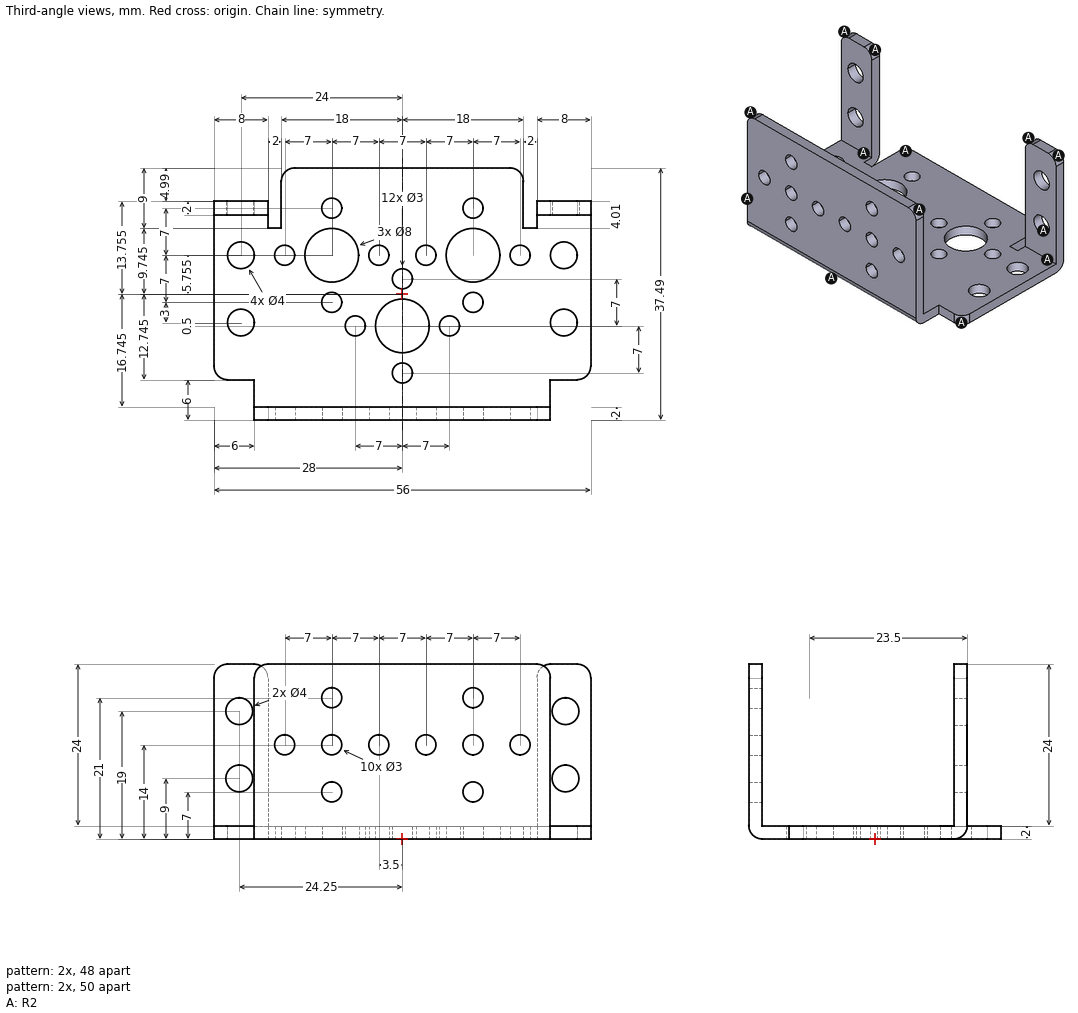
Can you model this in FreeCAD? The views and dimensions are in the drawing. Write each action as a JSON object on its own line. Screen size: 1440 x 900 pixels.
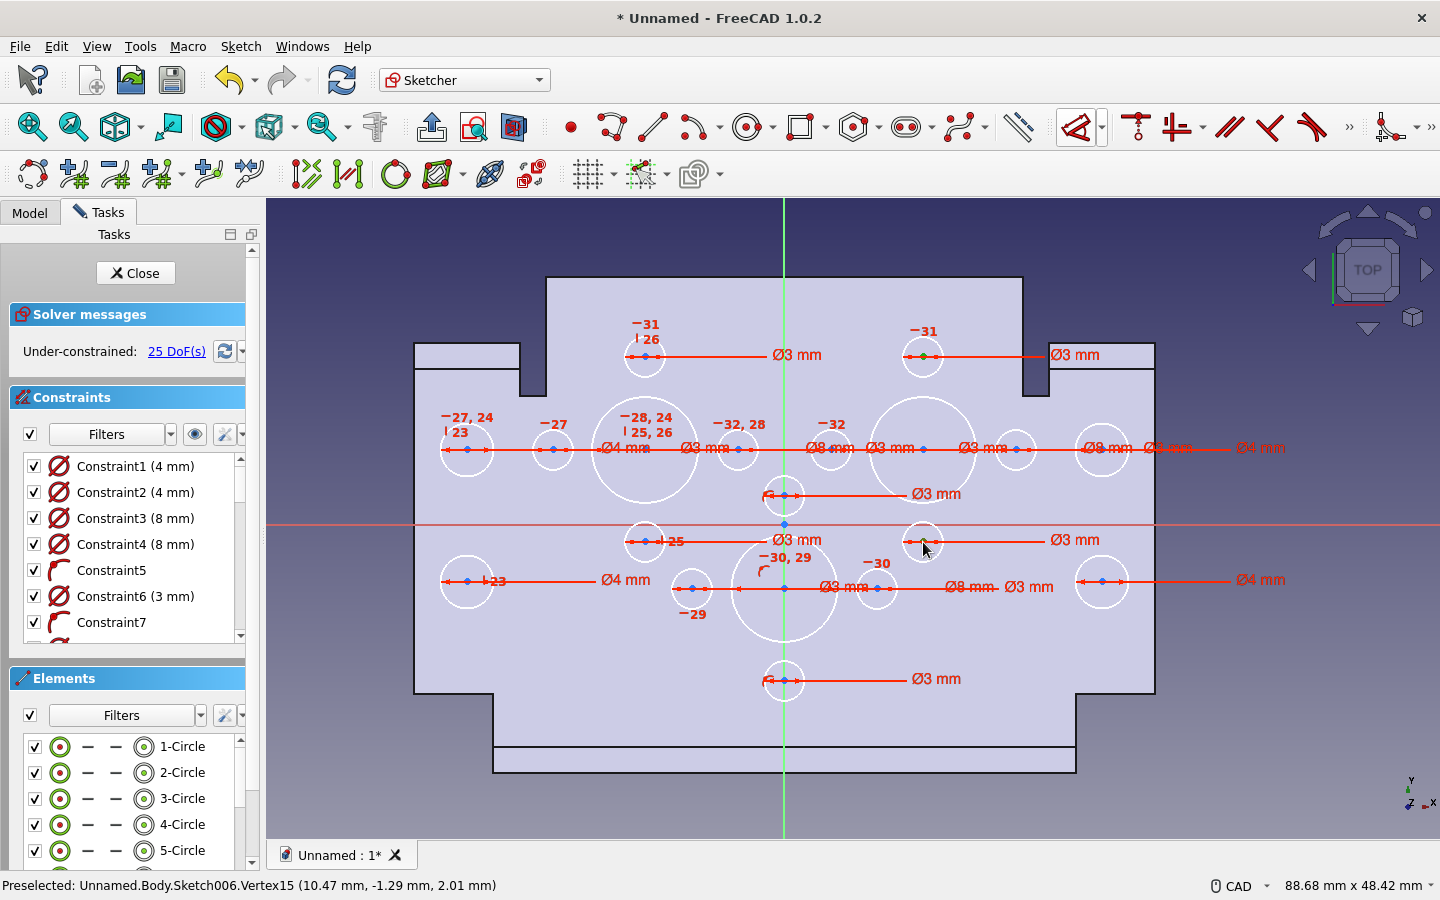
{"action": "key", "text": "v"}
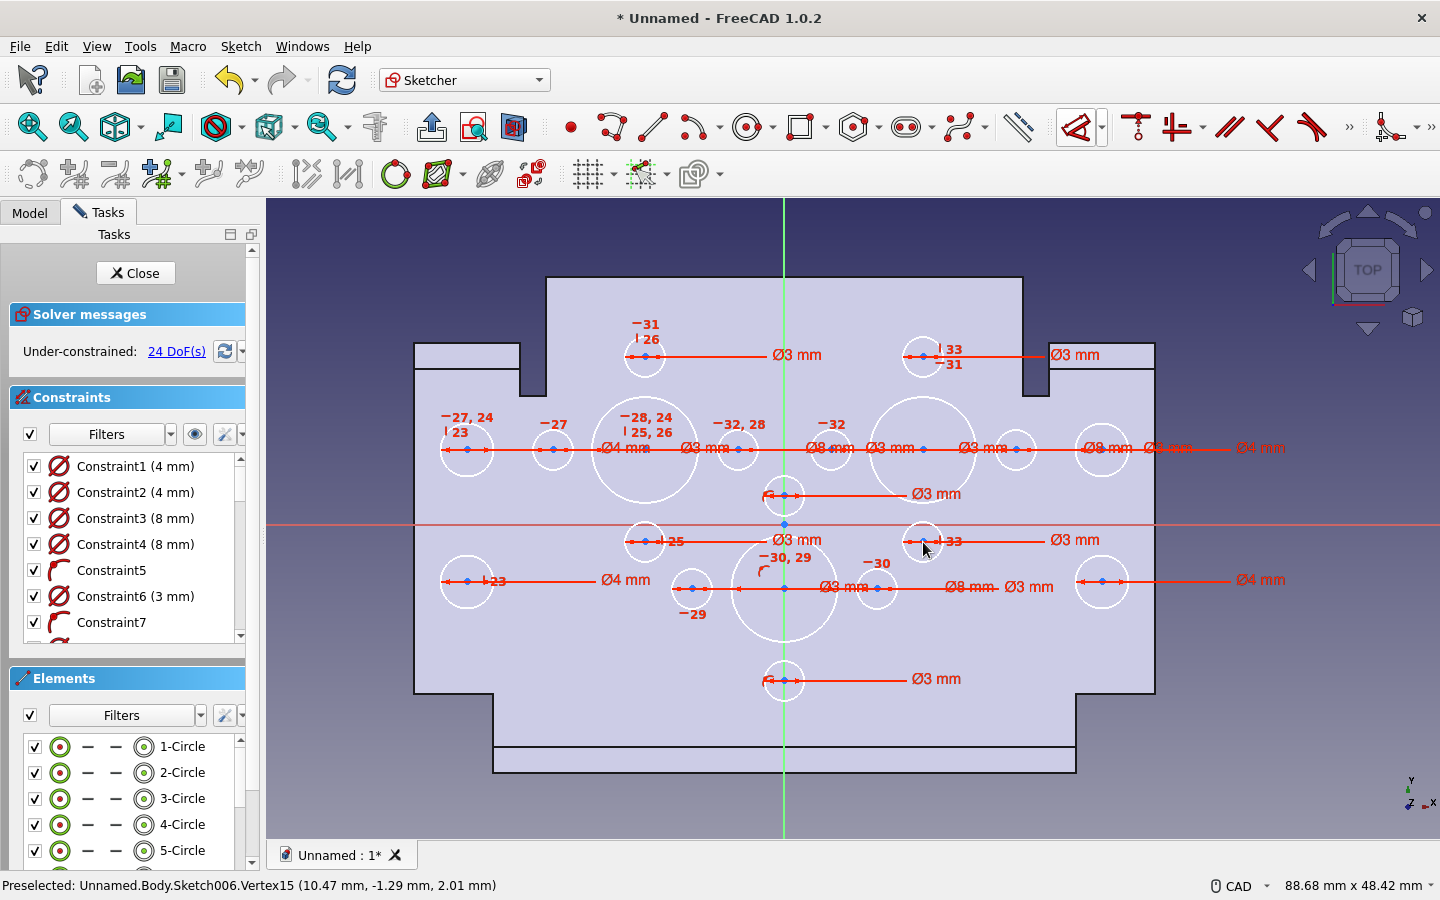
{"action": "left_click", "coordinate": [923, 542]}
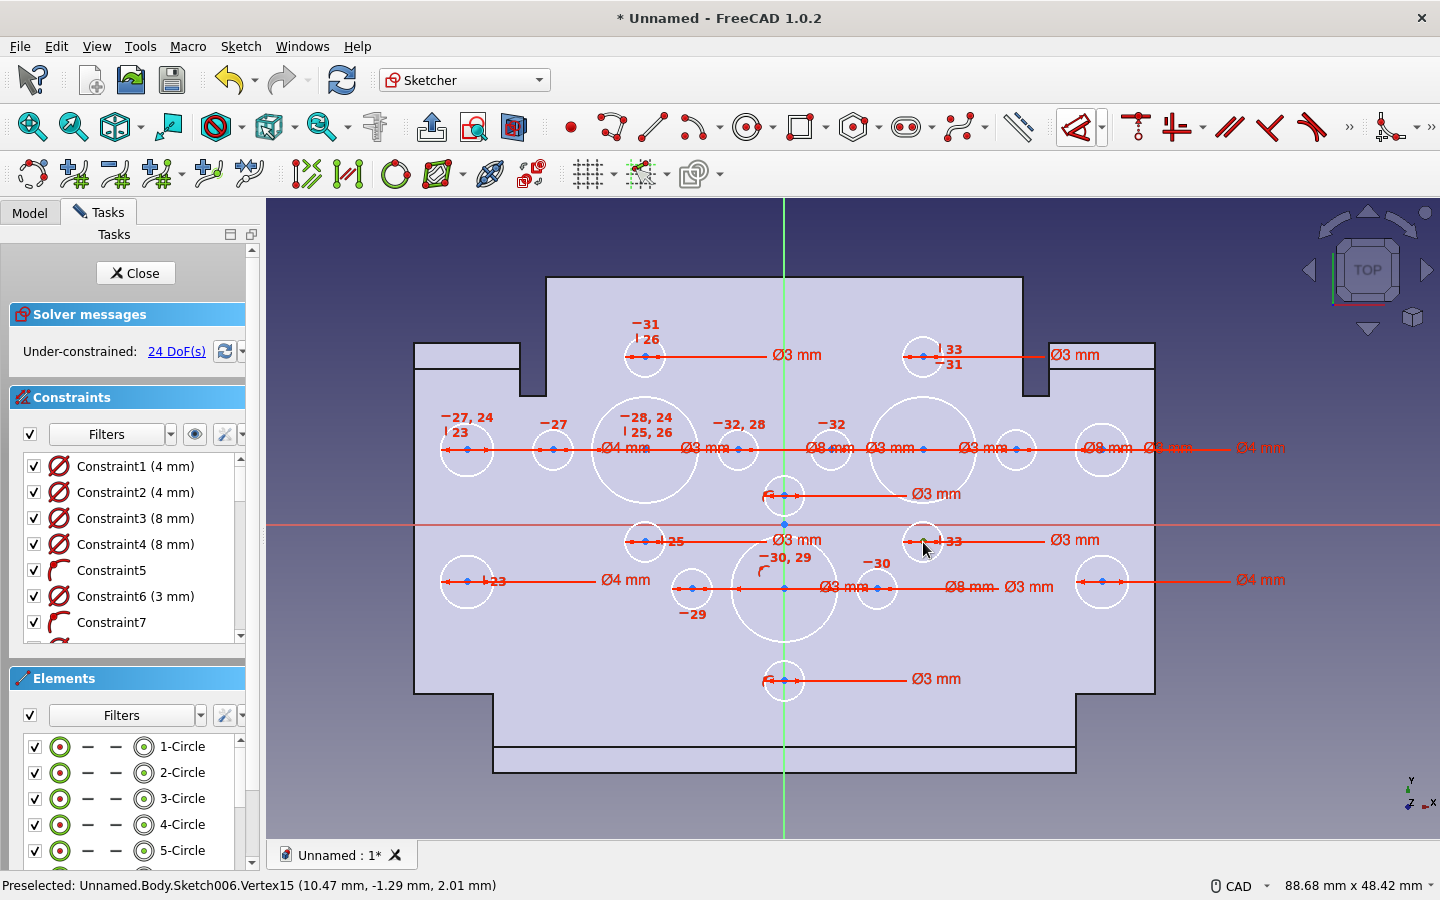
{"action": "left_click", "coordinate": [923, 450]}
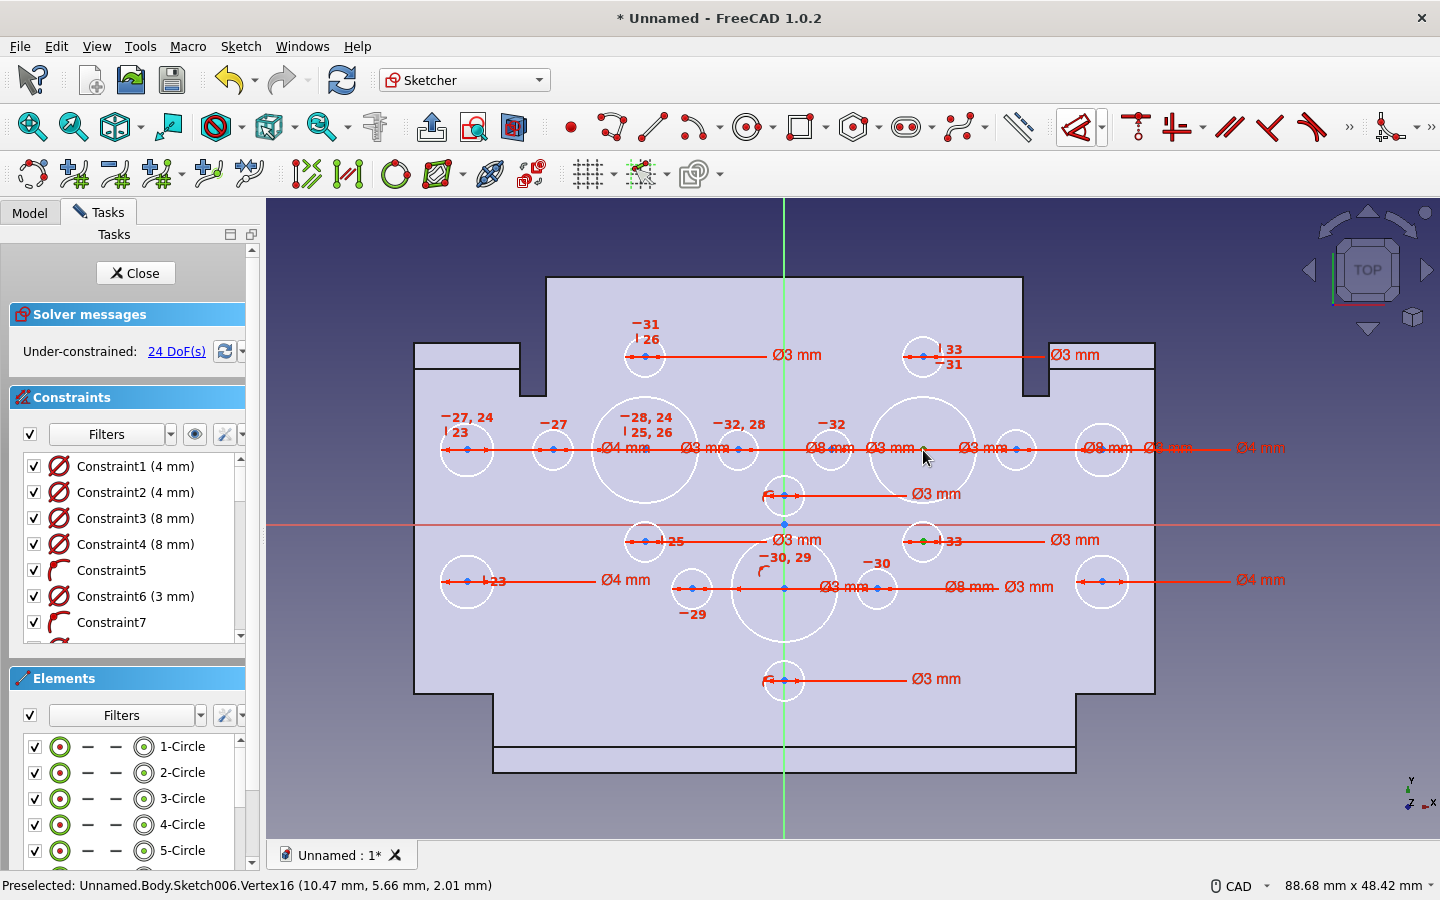
{"action": "key", "text": "v"}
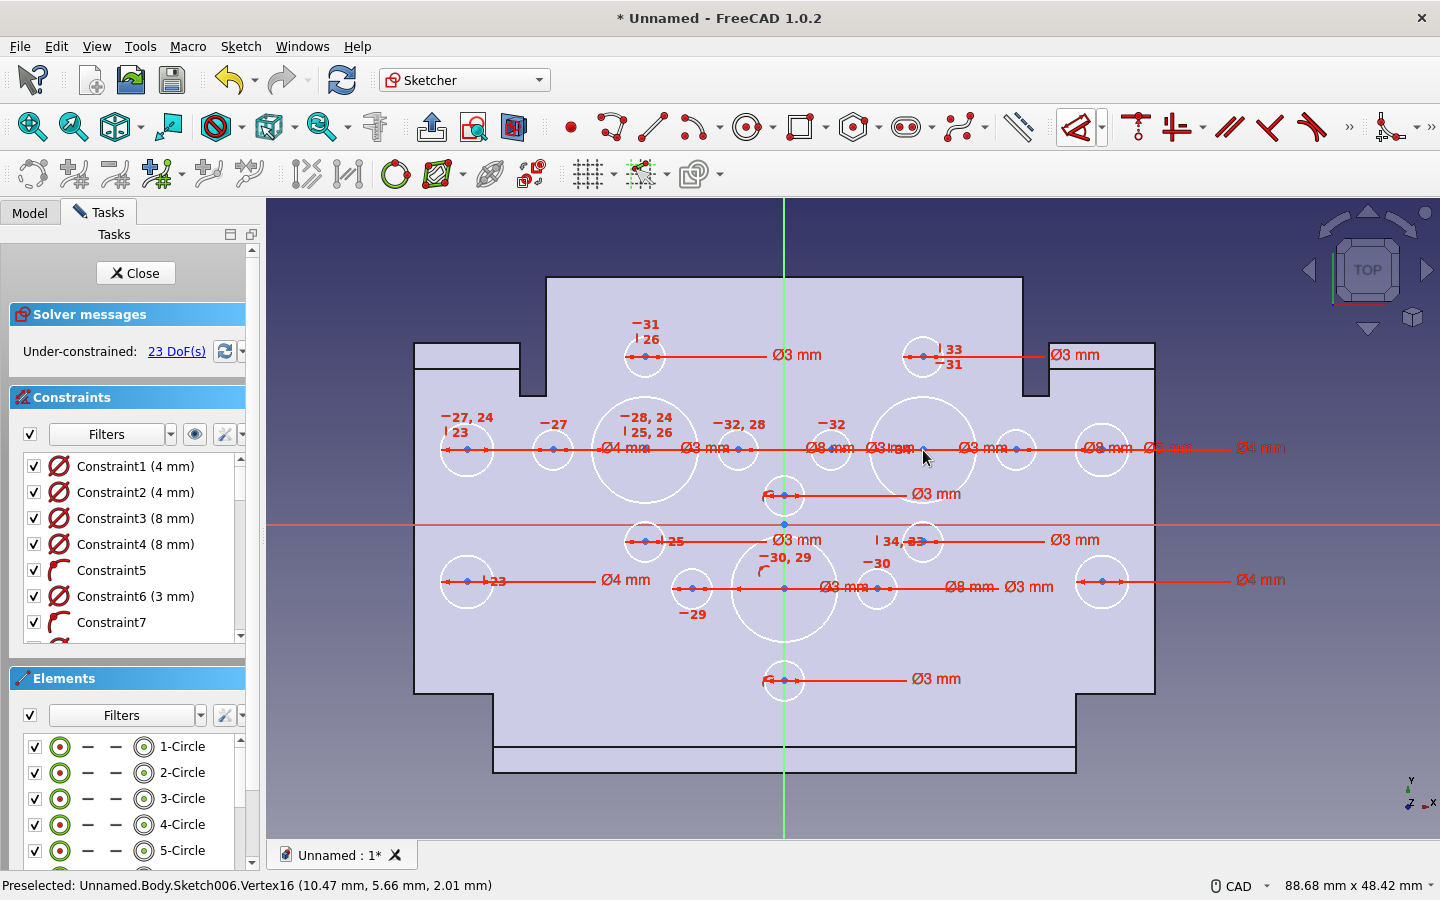
{"action": "left_click", "coordinate": [831, 450]}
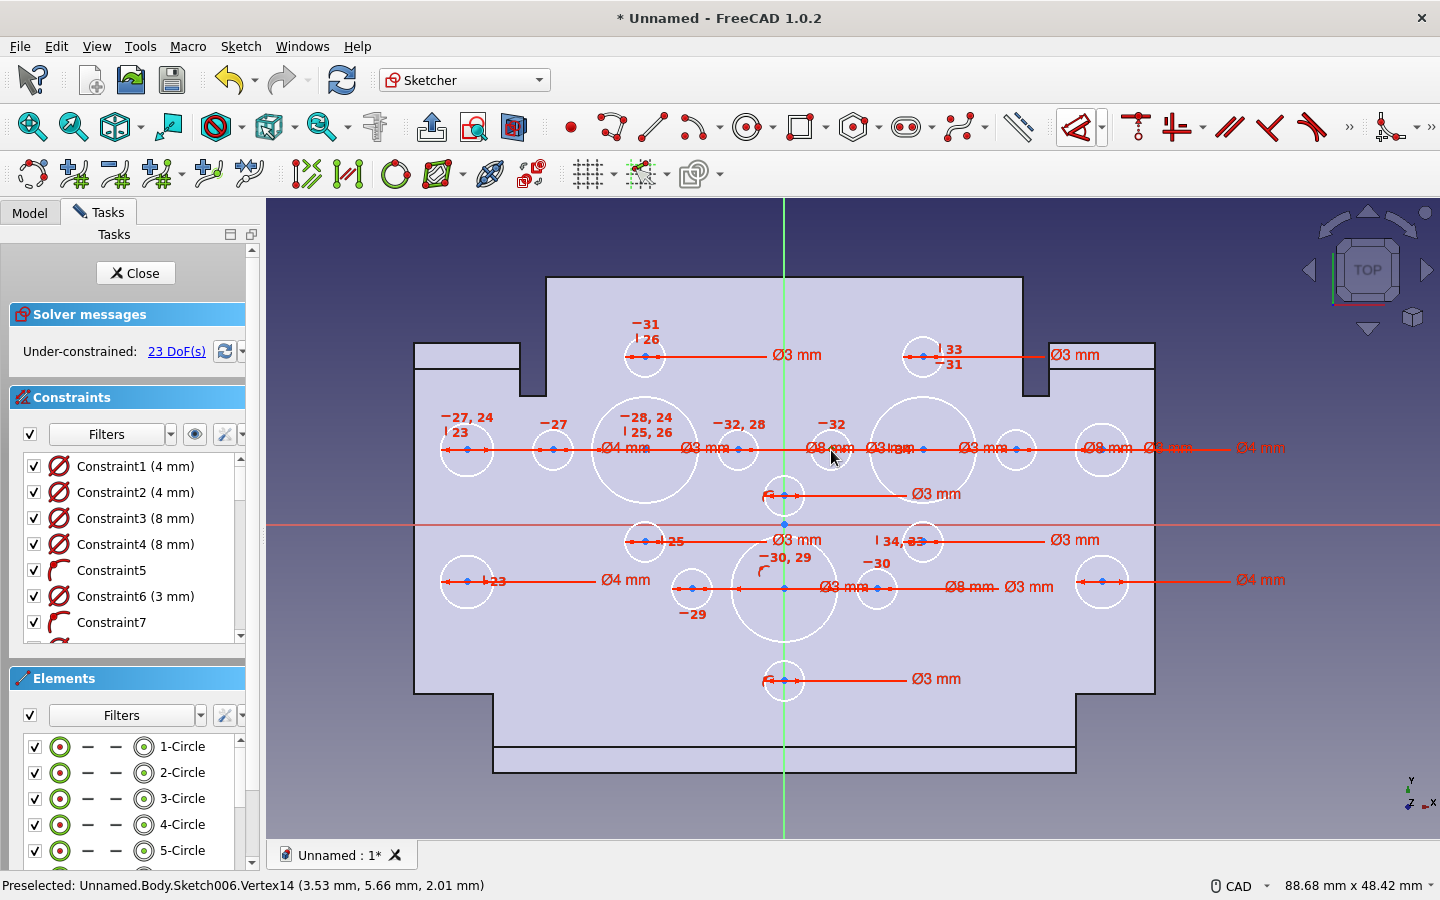
{"action": "left_click", "coordinate": [923, 450]}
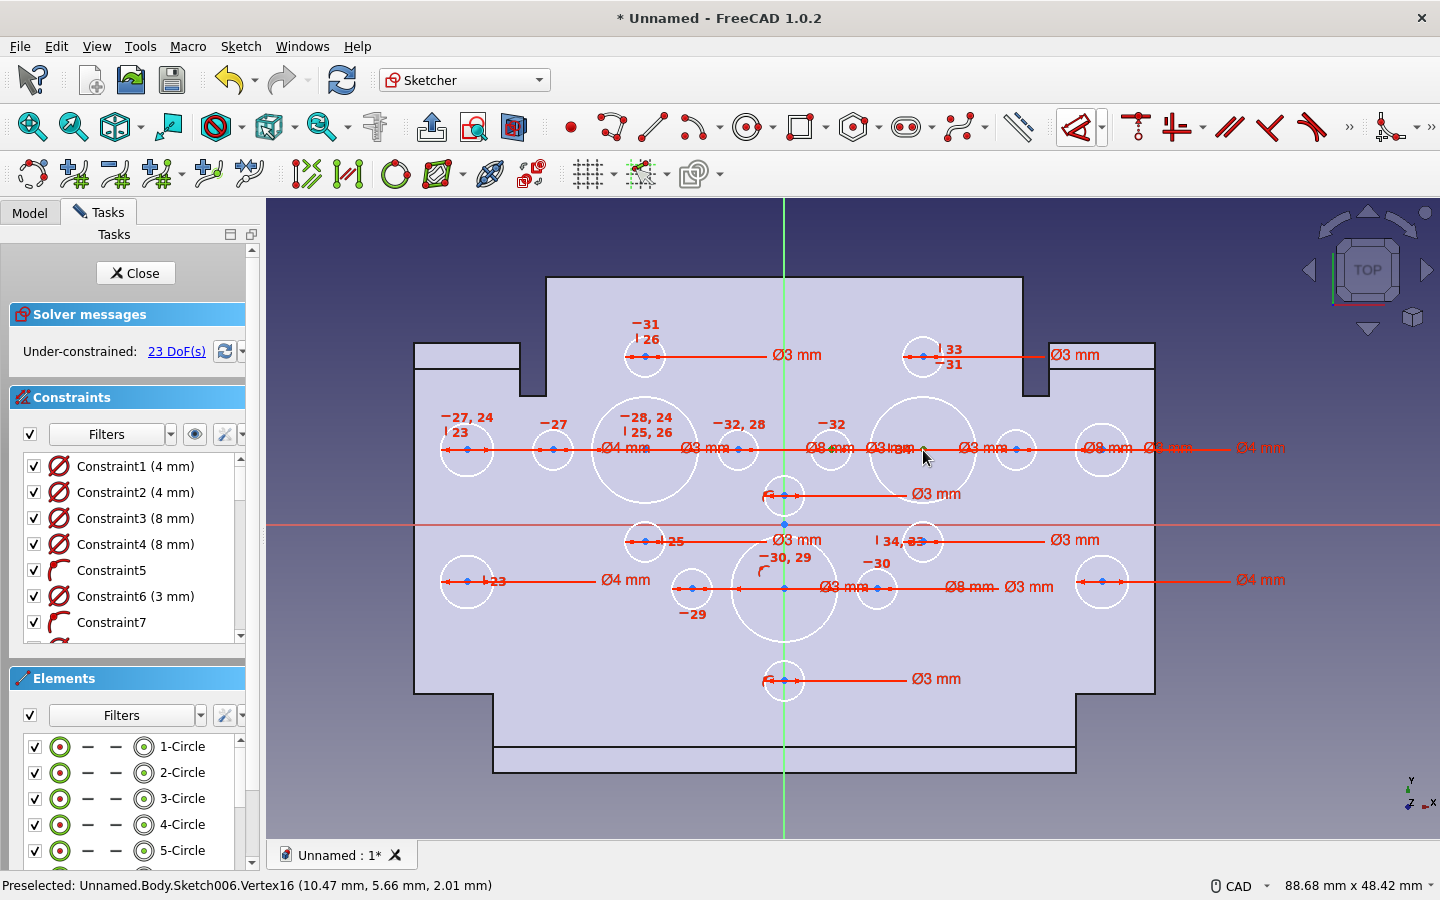
{"action": "key", "text": "h"}